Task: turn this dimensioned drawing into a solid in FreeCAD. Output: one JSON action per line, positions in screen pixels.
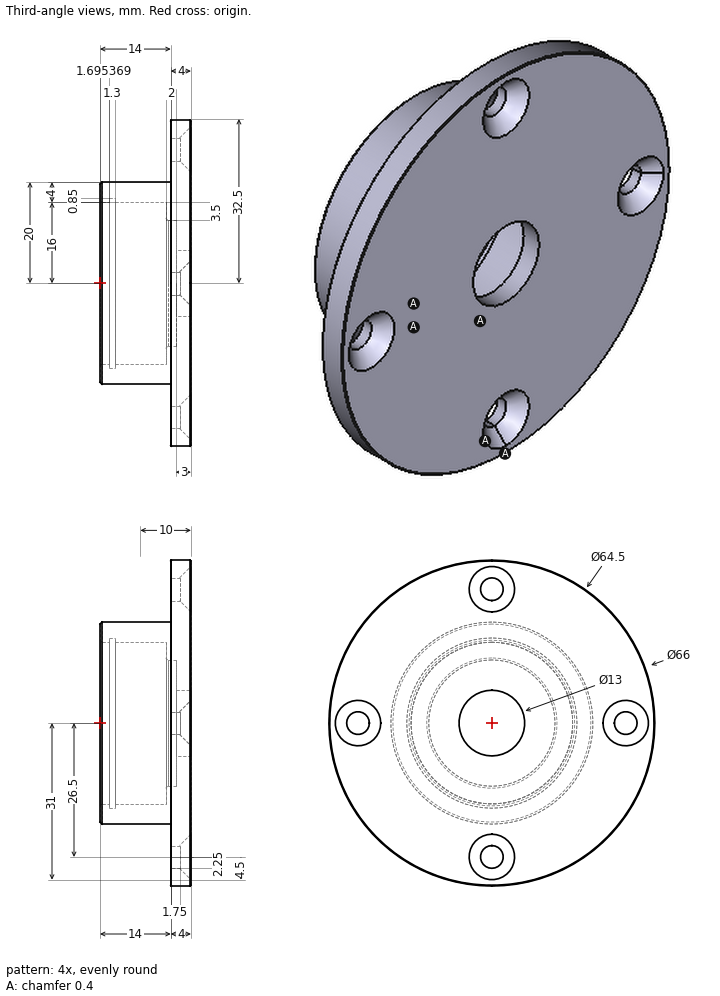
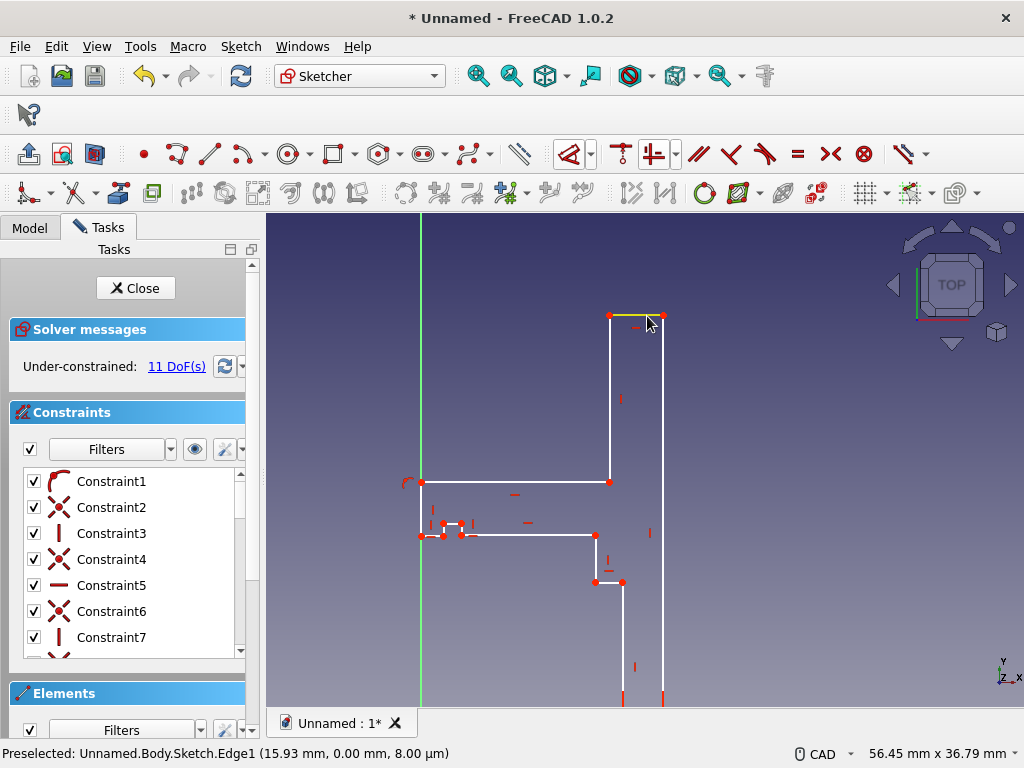
{"action": "left_click", "coordinate": [647, 315]}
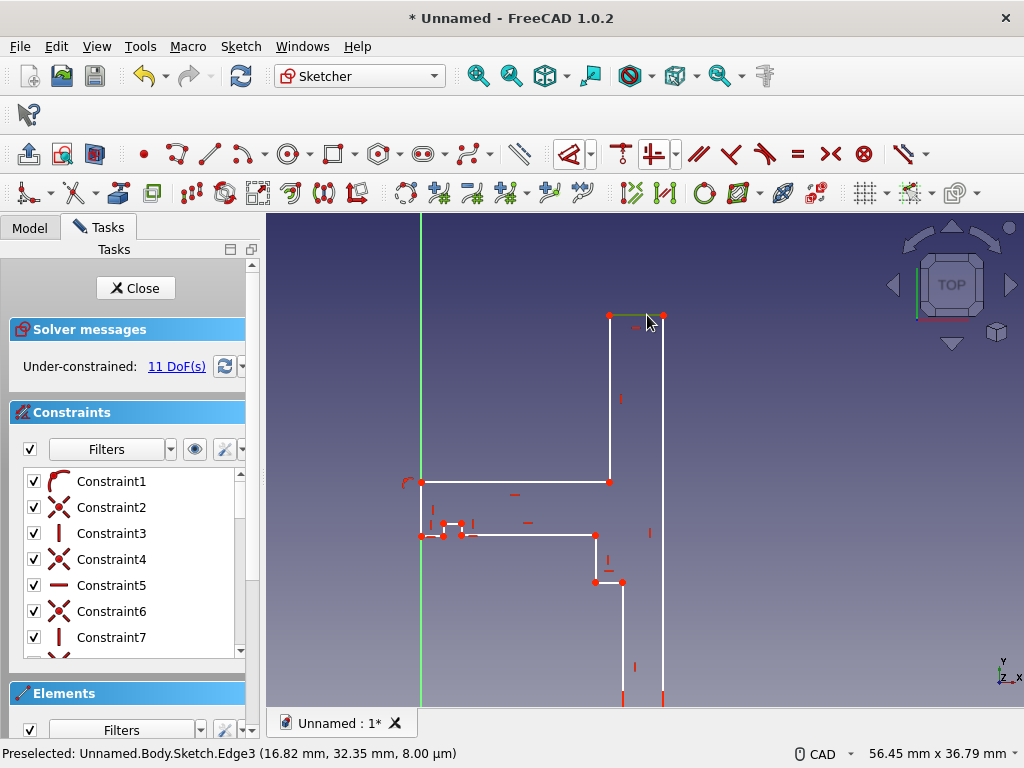
{"action": "left_click", "coordinate": [590, 154]}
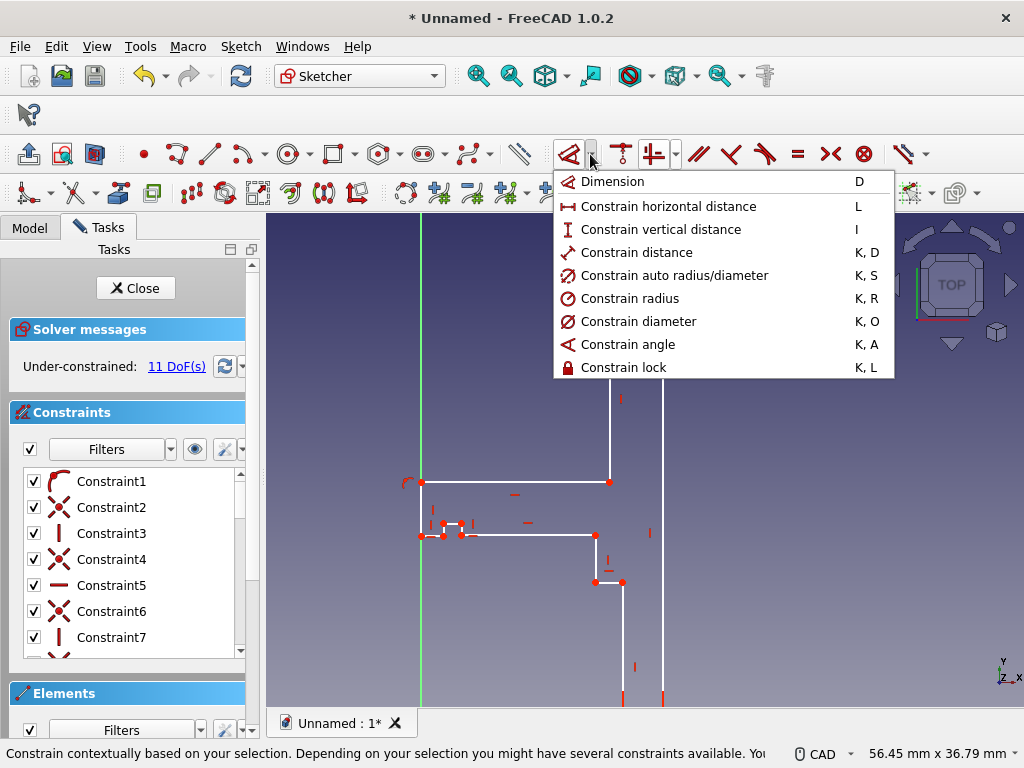
{"action": "left_click", "coordinate": [724, 206]}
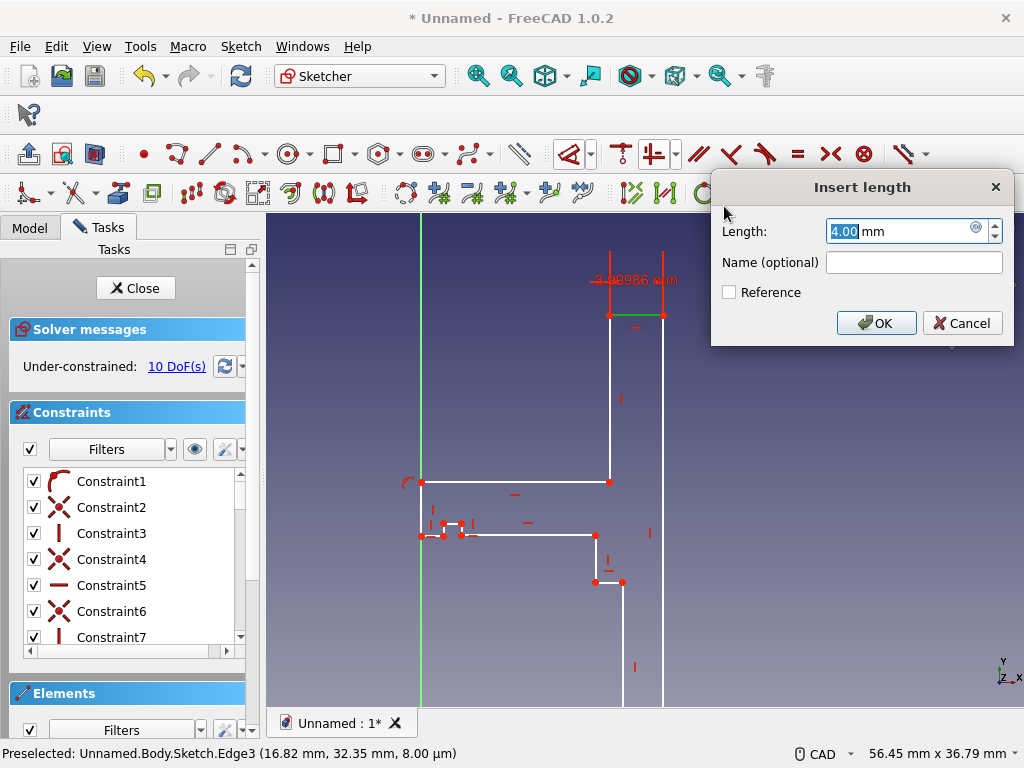
{"action": "type", "text": "4"}
{"action": "key", "text": "Return"}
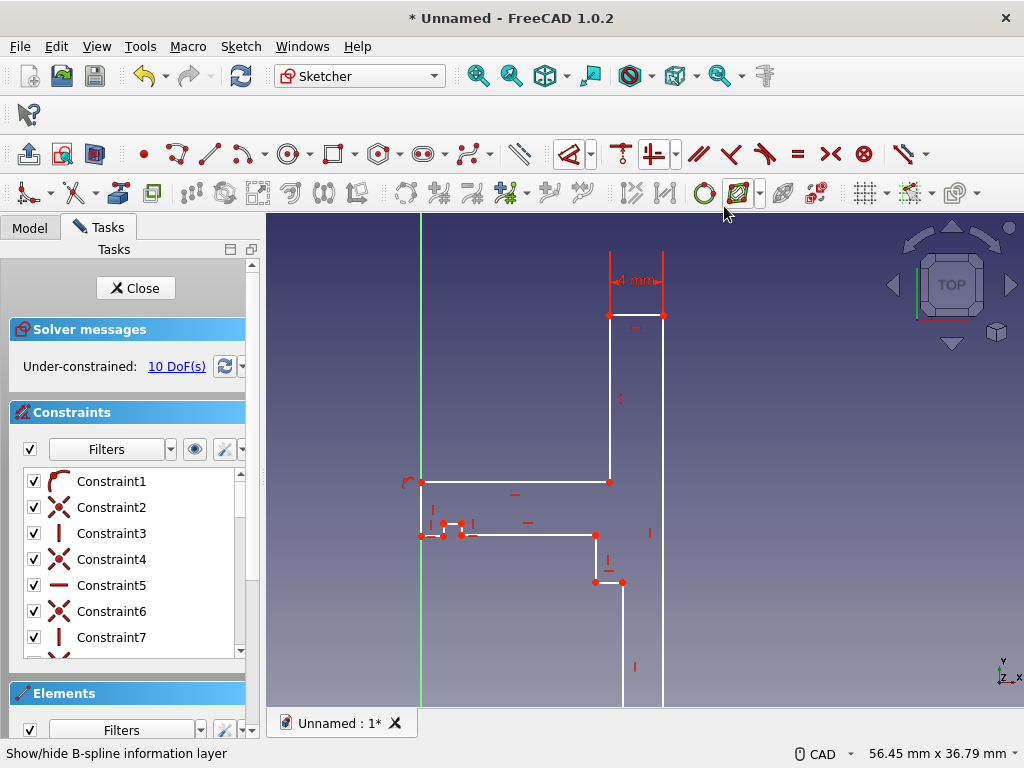
{"action": "left_click", "coordinate": [421, 499]}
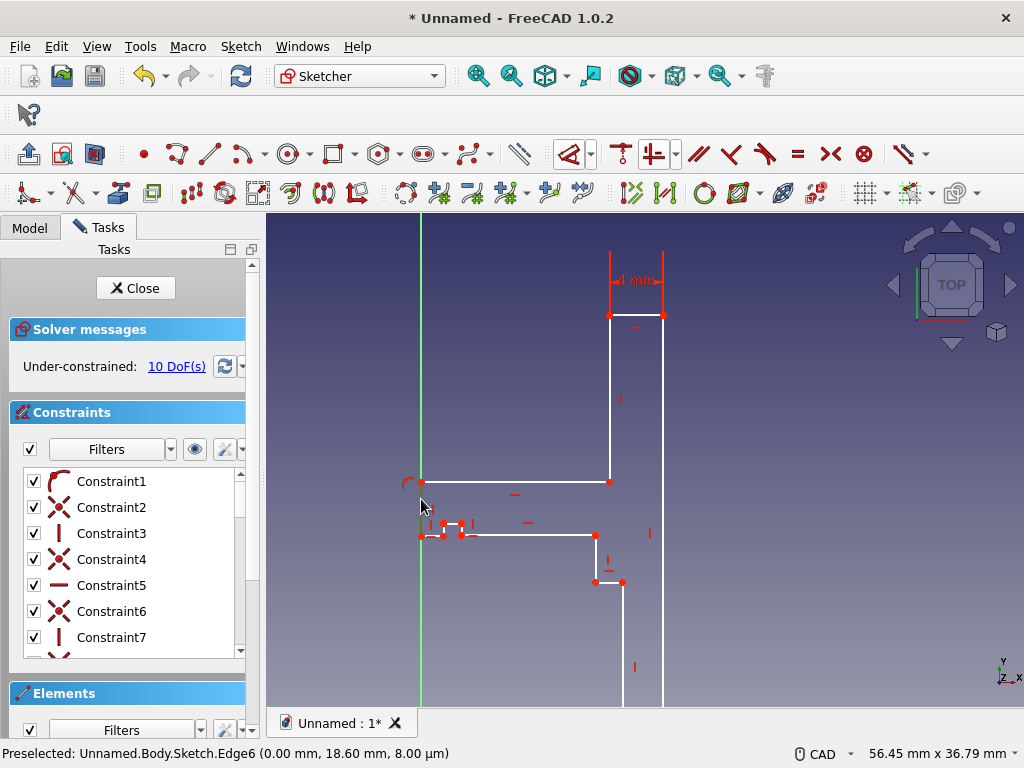
{"action": "left_click", "coordinate": [590, 154]}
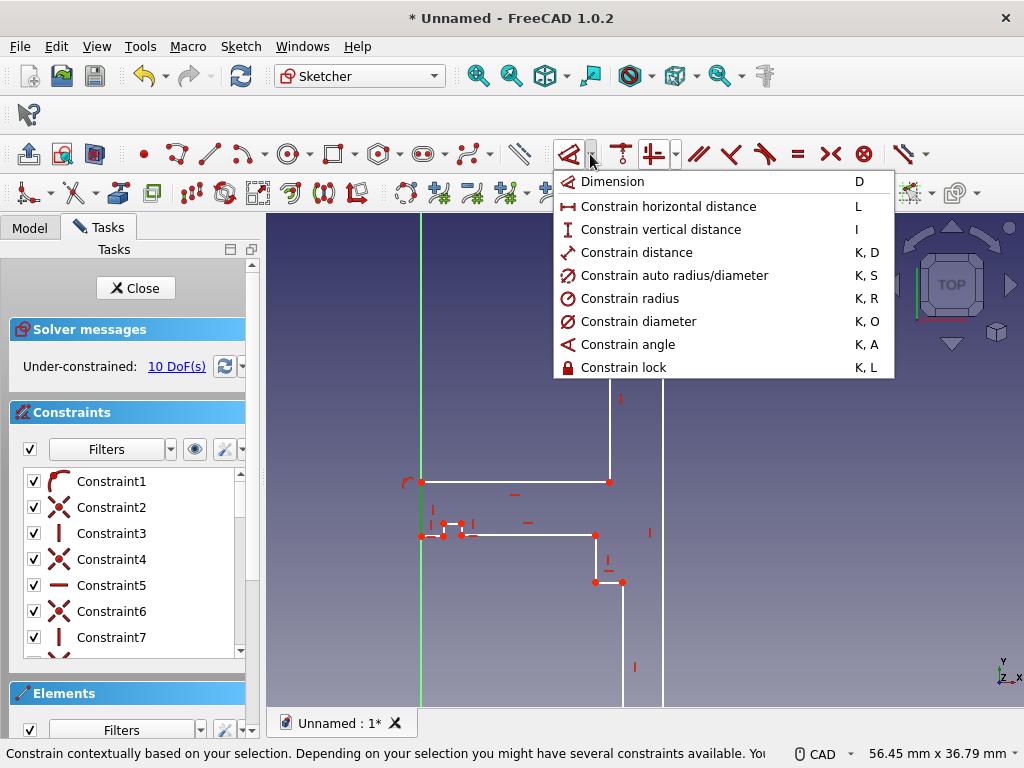
{"action": "left_click", "coordinate": [724, 230]}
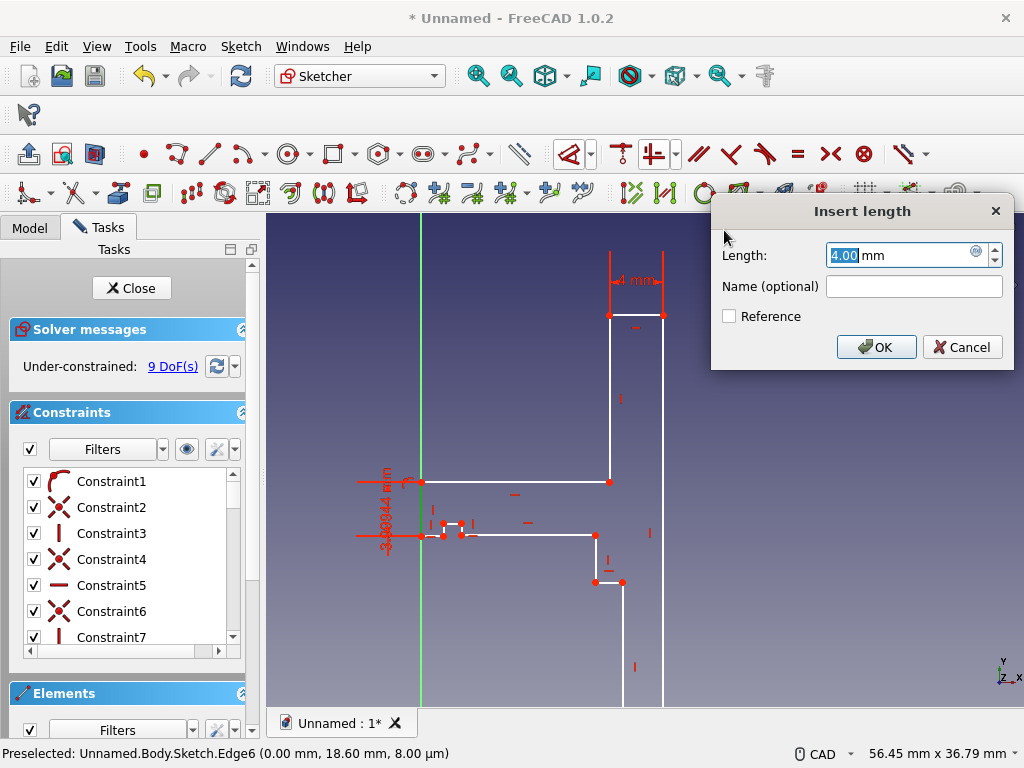
{"action": "type", "text": "4"}
{"action": "key", "text": "Return"}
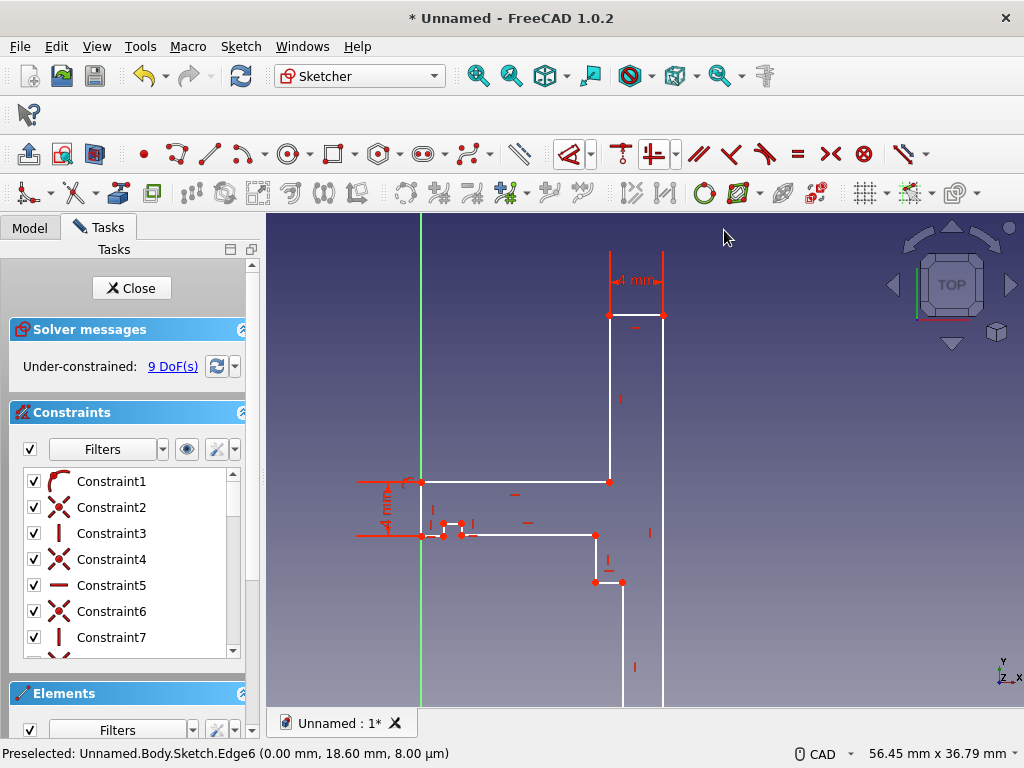
{"action": "scroll", "coordinate": [607, 583], "scroll_direction": "up", "scroll_amount": 2}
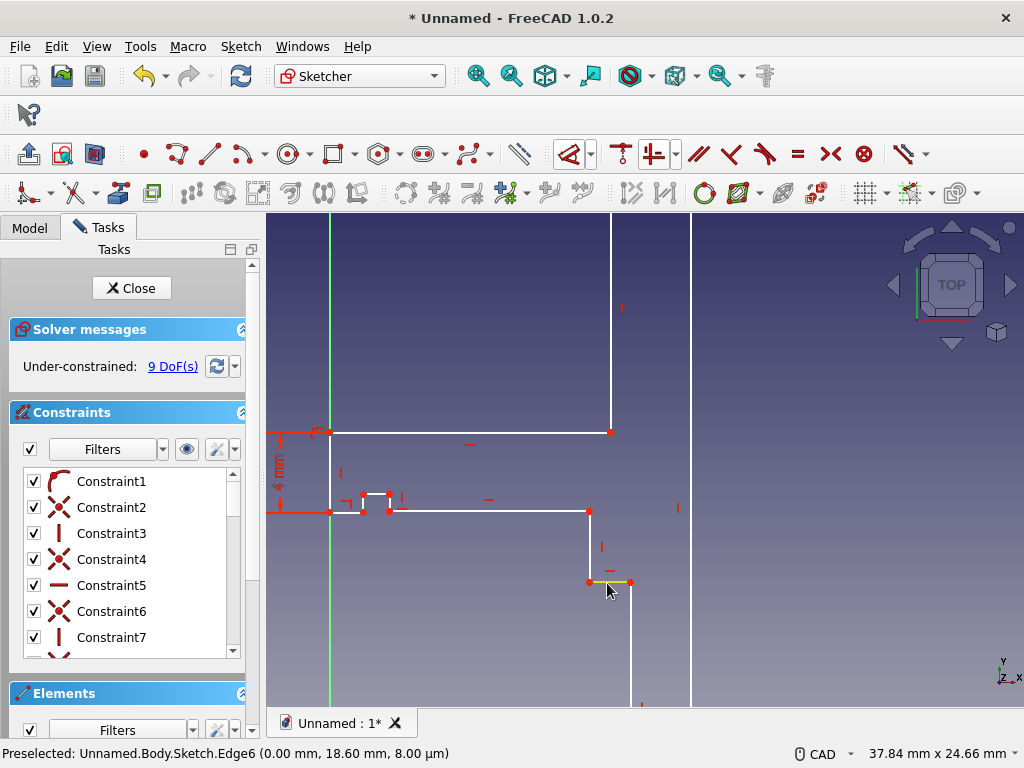
{"action": "left_click", "coordinate": [606, 582]}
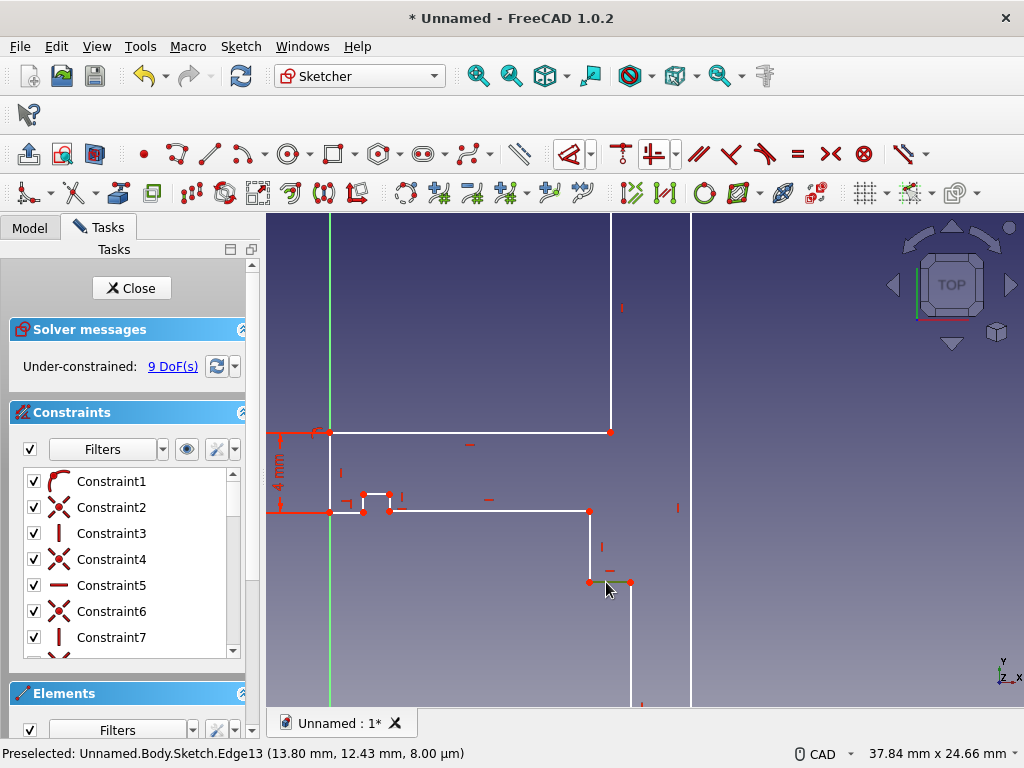
{"action": "key", "text": "l"}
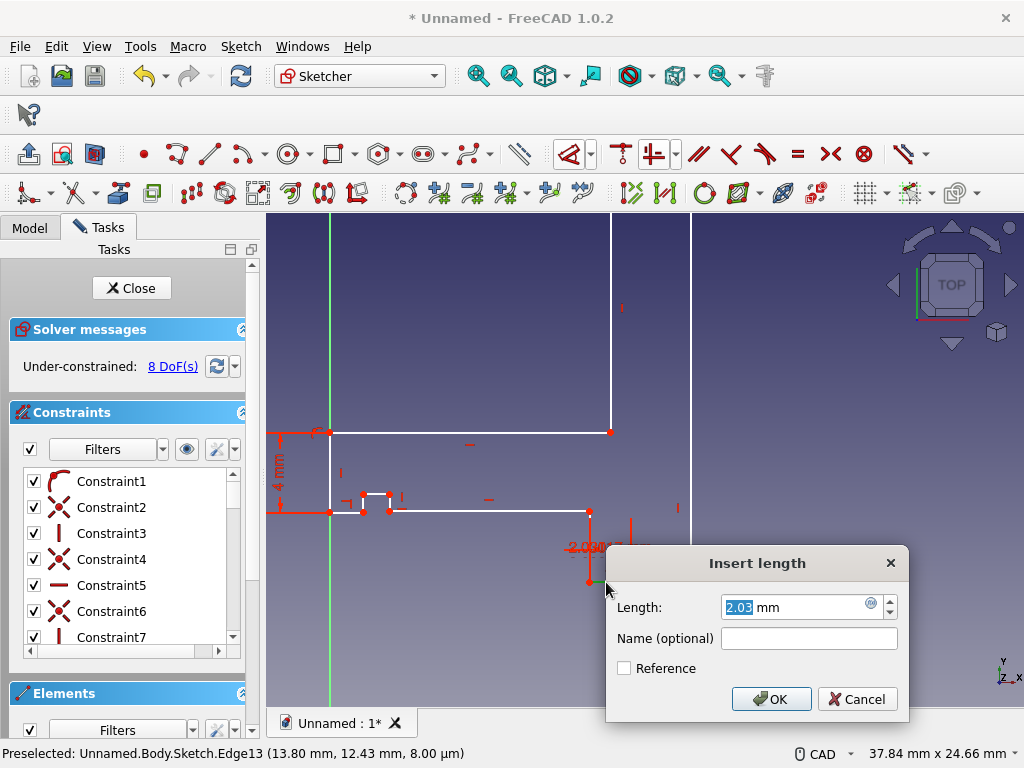
{"action": "type", "text": "2"}
{"action": "key", "text": "Return"}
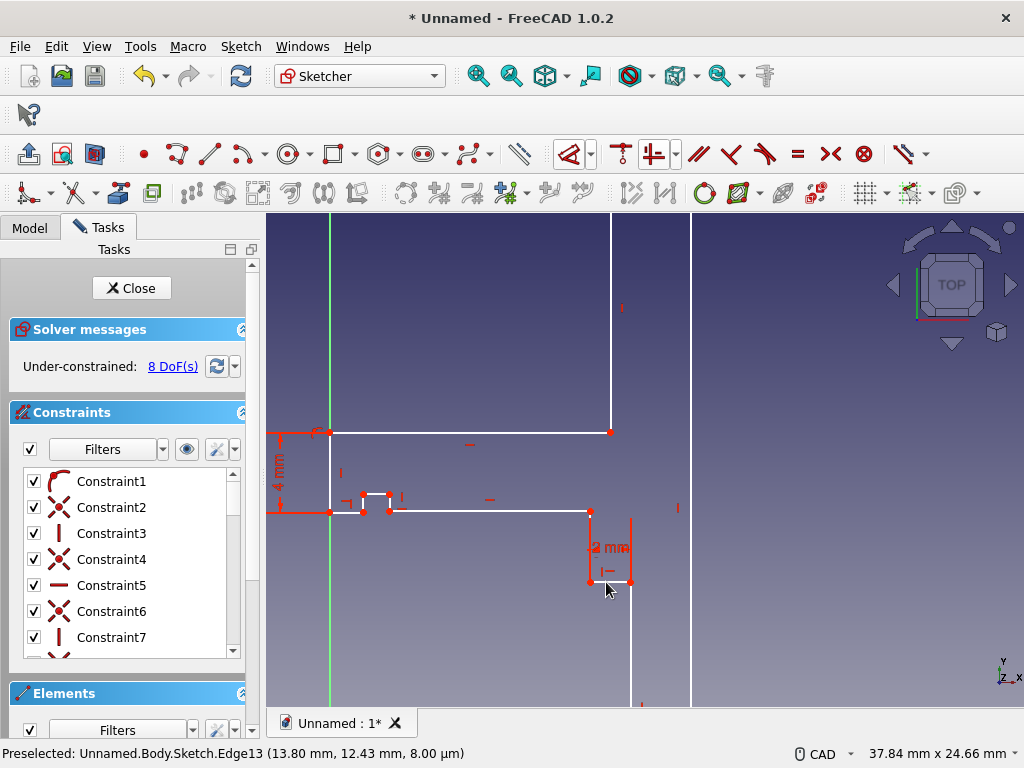
{"action": "left_click", "coordinate": [526, 433]}